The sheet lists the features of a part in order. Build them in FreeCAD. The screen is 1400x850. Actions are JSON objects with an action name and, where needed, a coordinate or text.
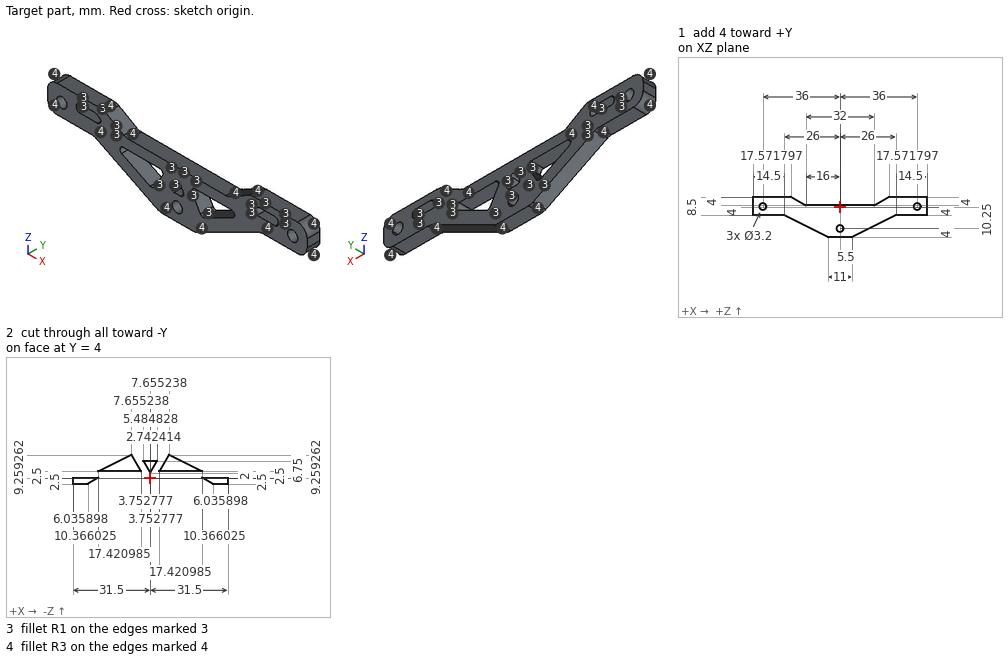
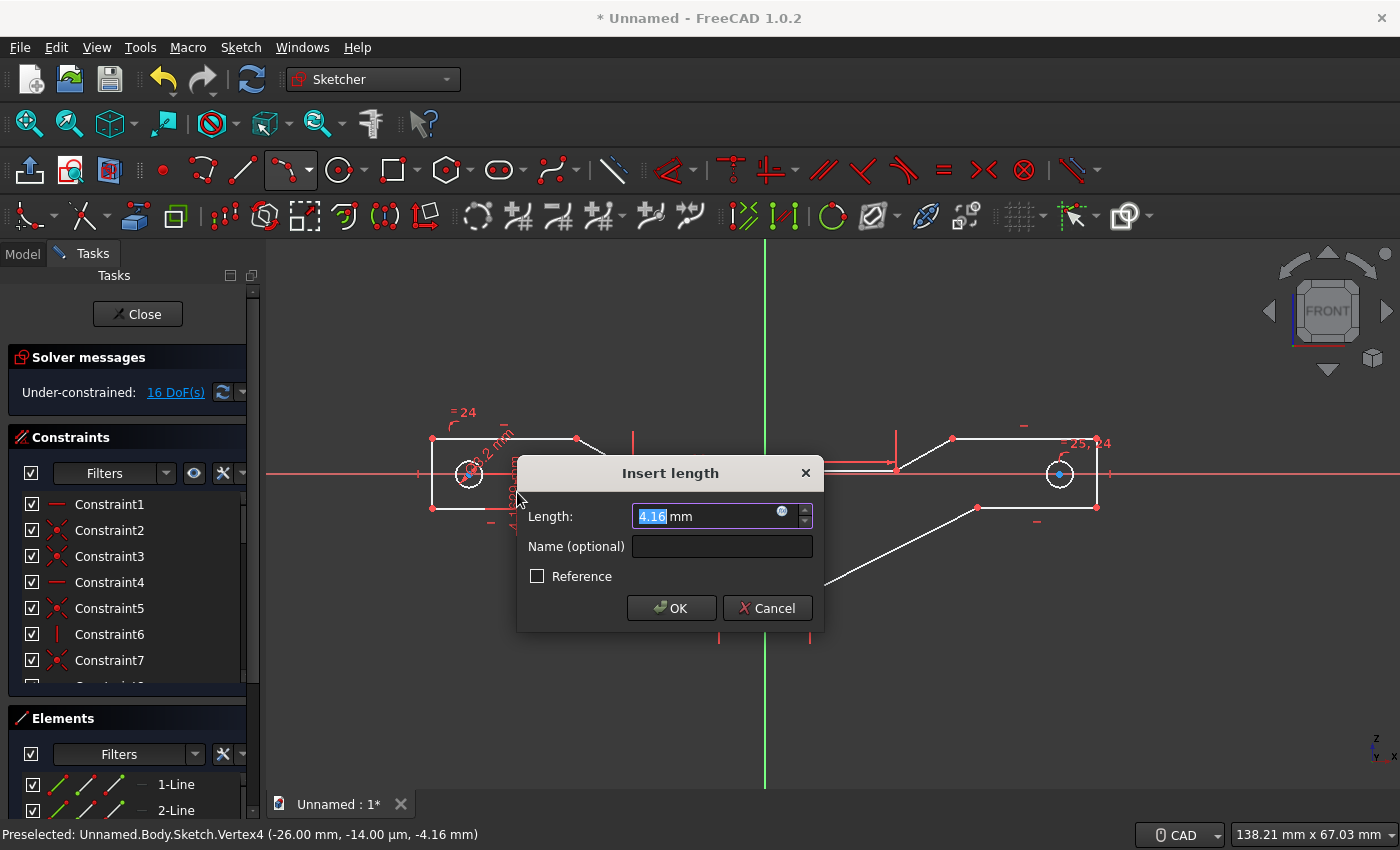
{"action": "type", "text": "4"}
{"action": "key", "text": "Return"}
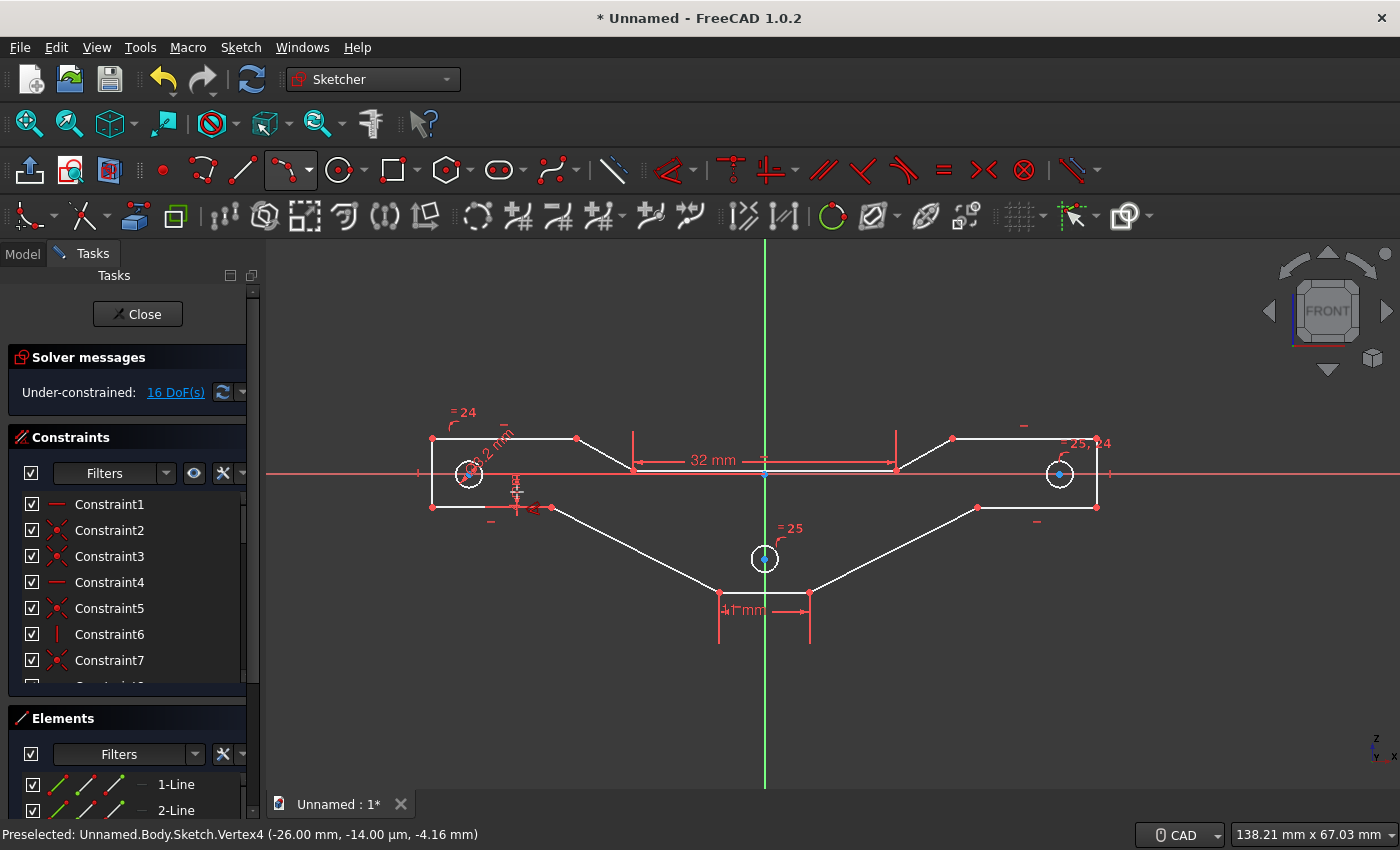
{"action": "left_click", "coordinate": [1097, 508]}
{"action": "left_click", "coordinate": [1131, 491]}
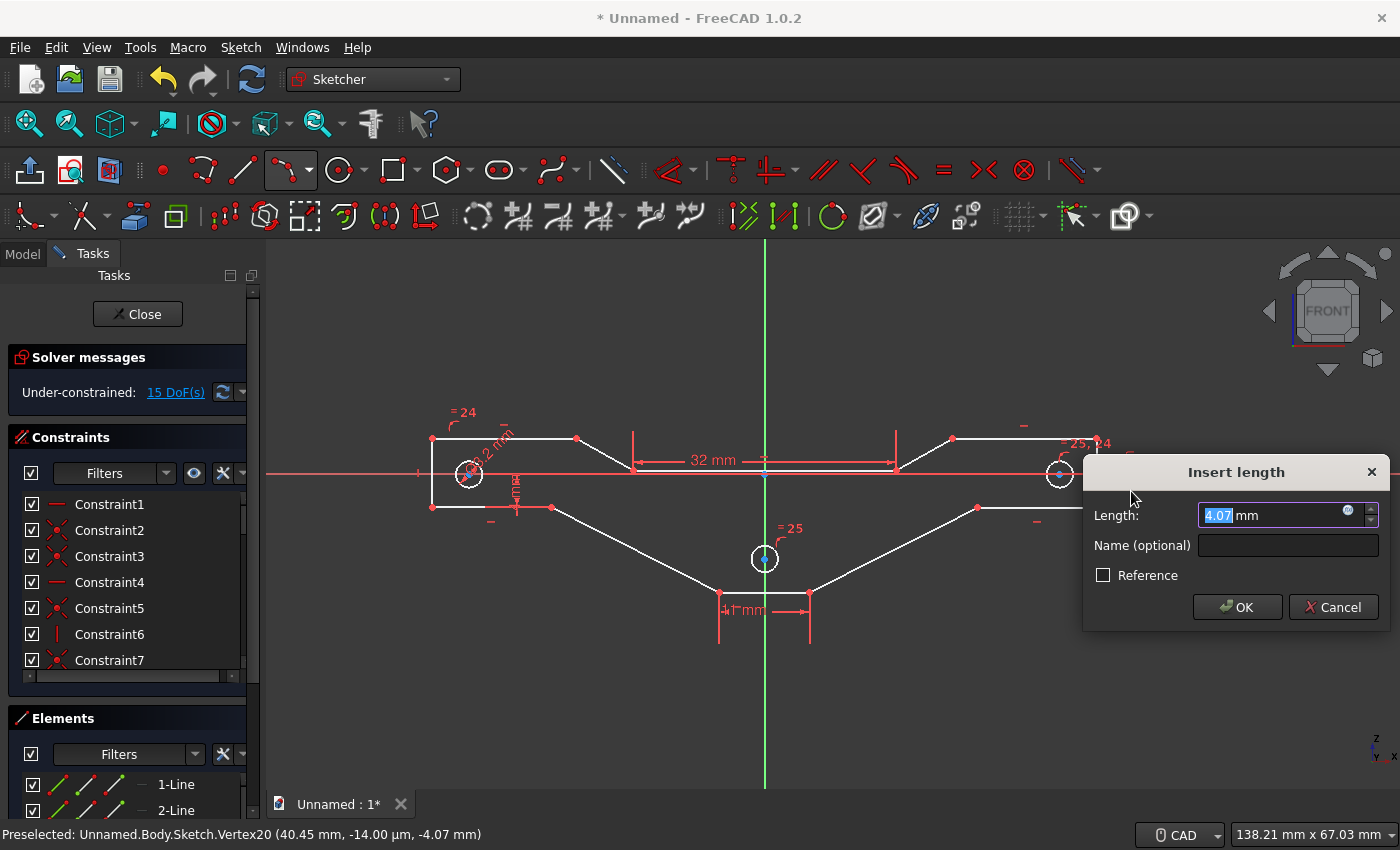
{"action": "type", "text": "4"}
{"action": "key", "text": "Return"}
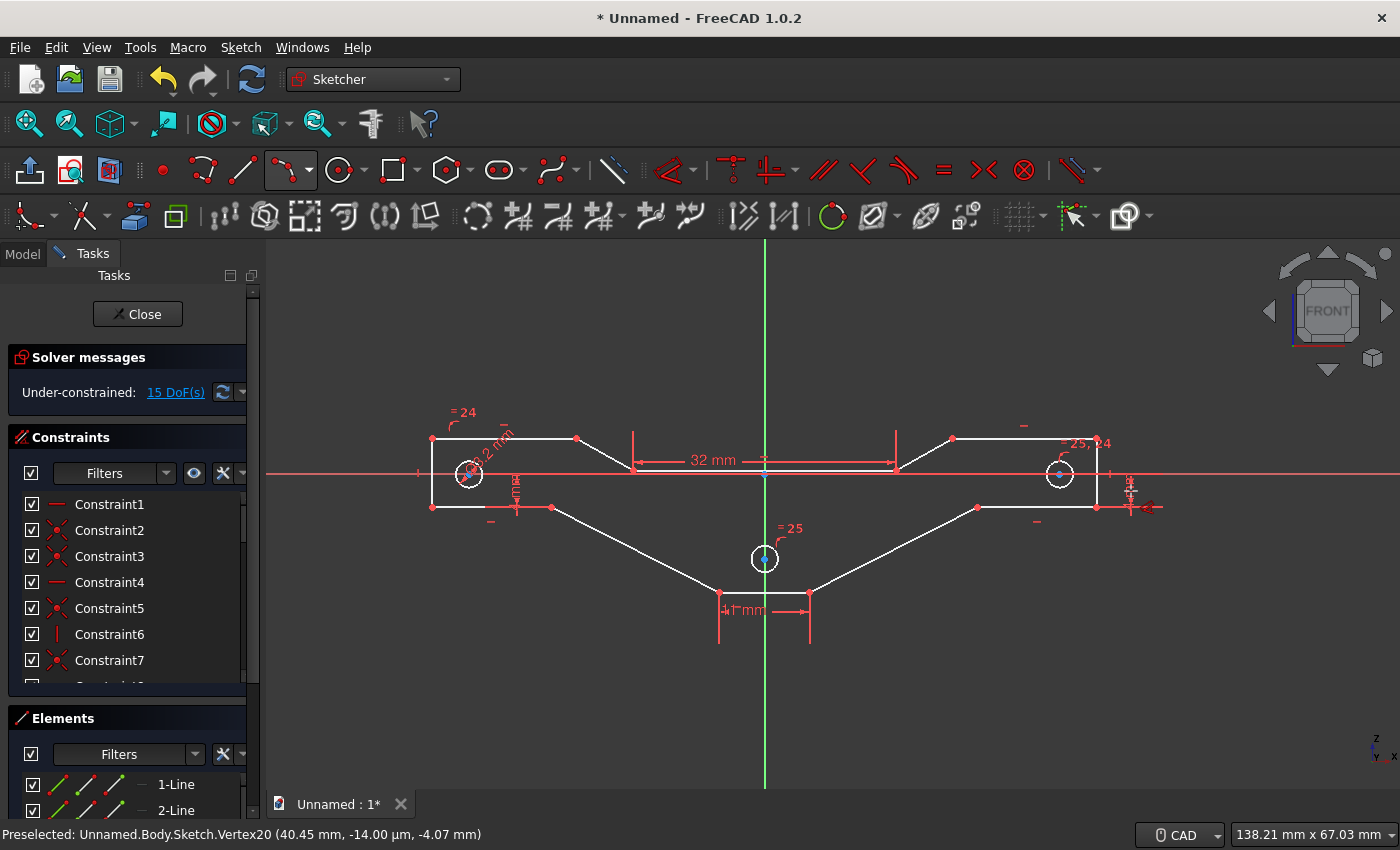
{"action": "left_click", "coordinate": [594, 448]}
{"action": "left_click", "coordinate": [787, 455]}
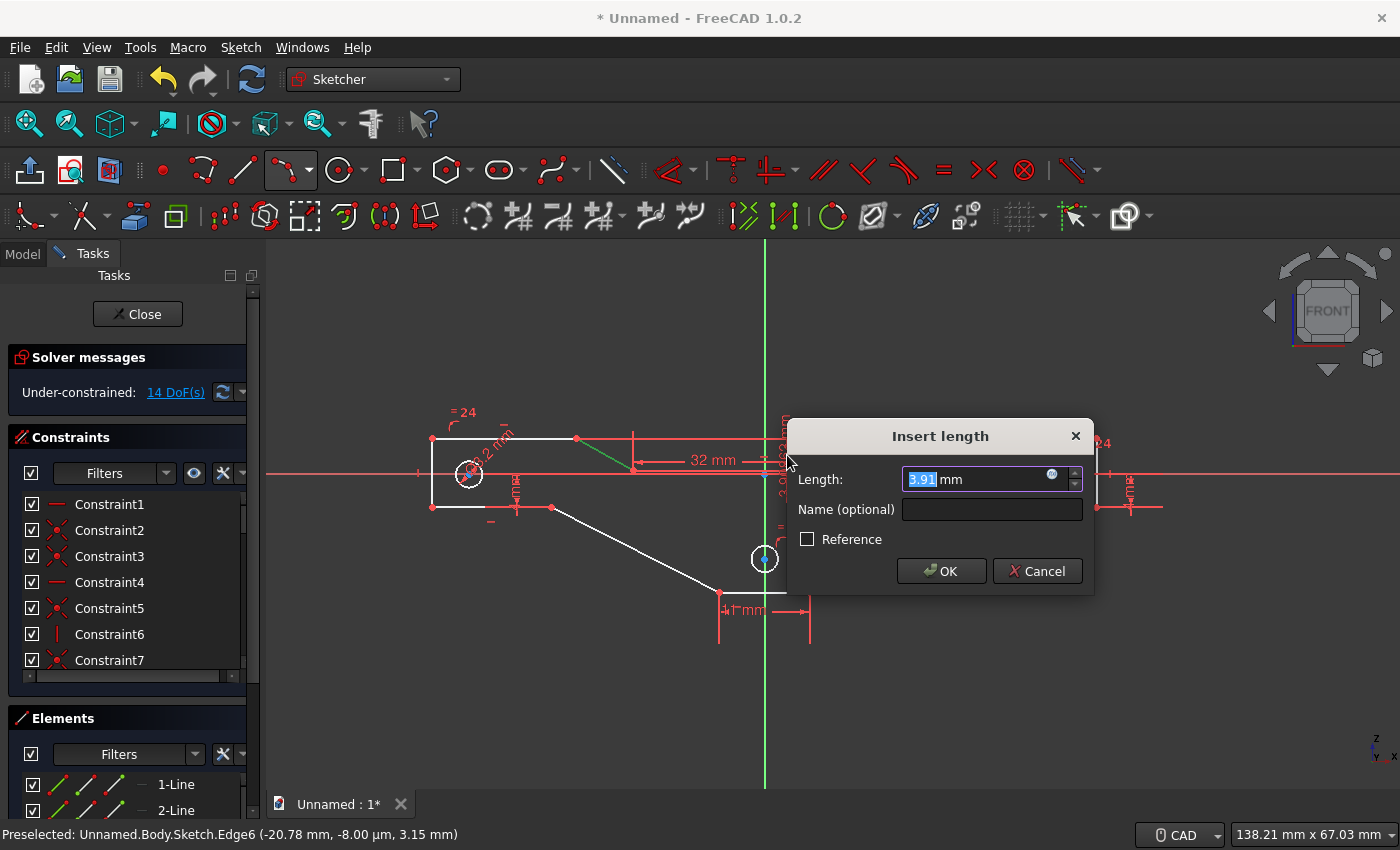
{"action": "type", "text": "4"}
{"action": "key", "text": "Return"}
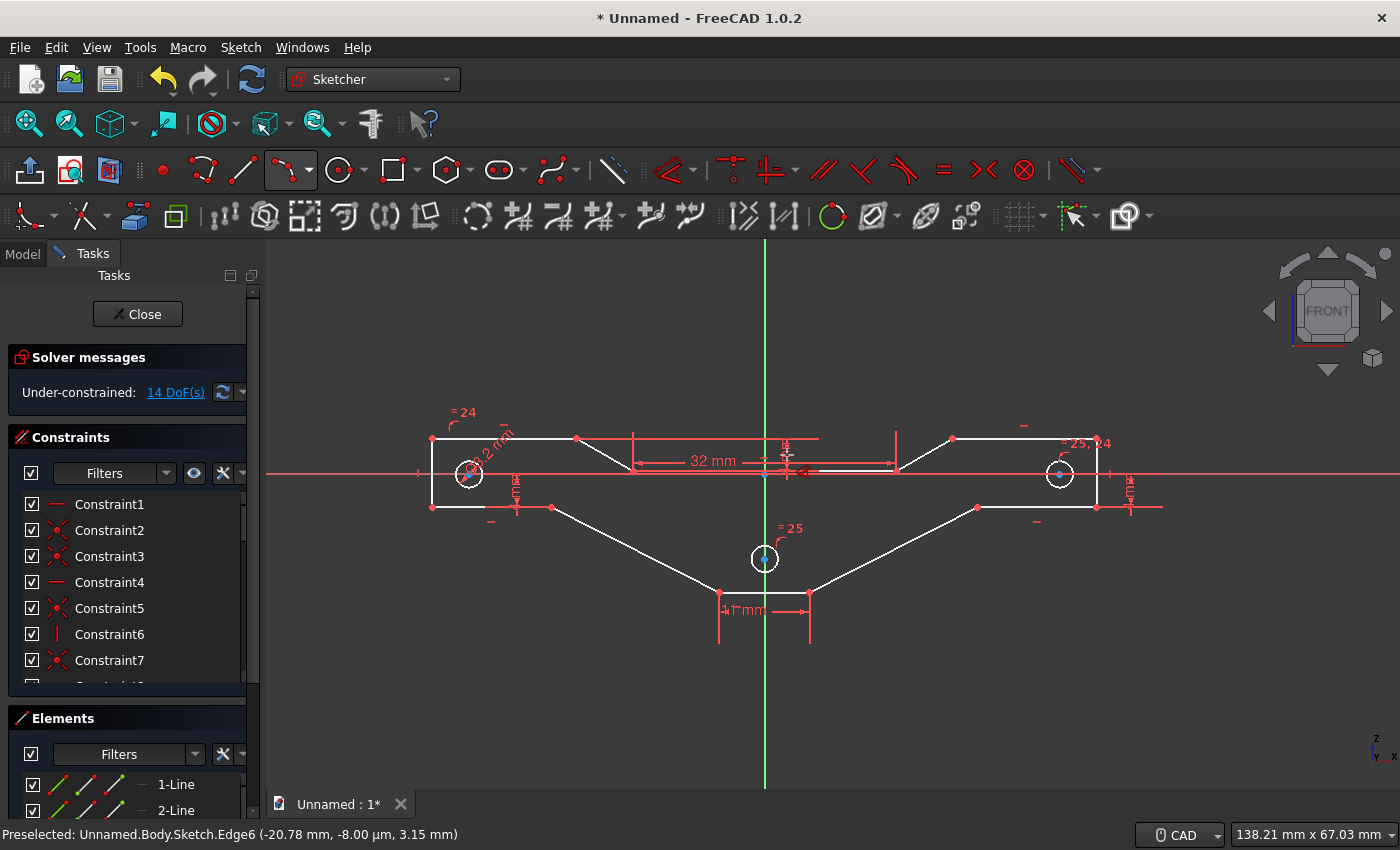
{"action": "left_click", "coordinate": [913, 462]}
{"action": "left_click", "coordinate": [987, 455]}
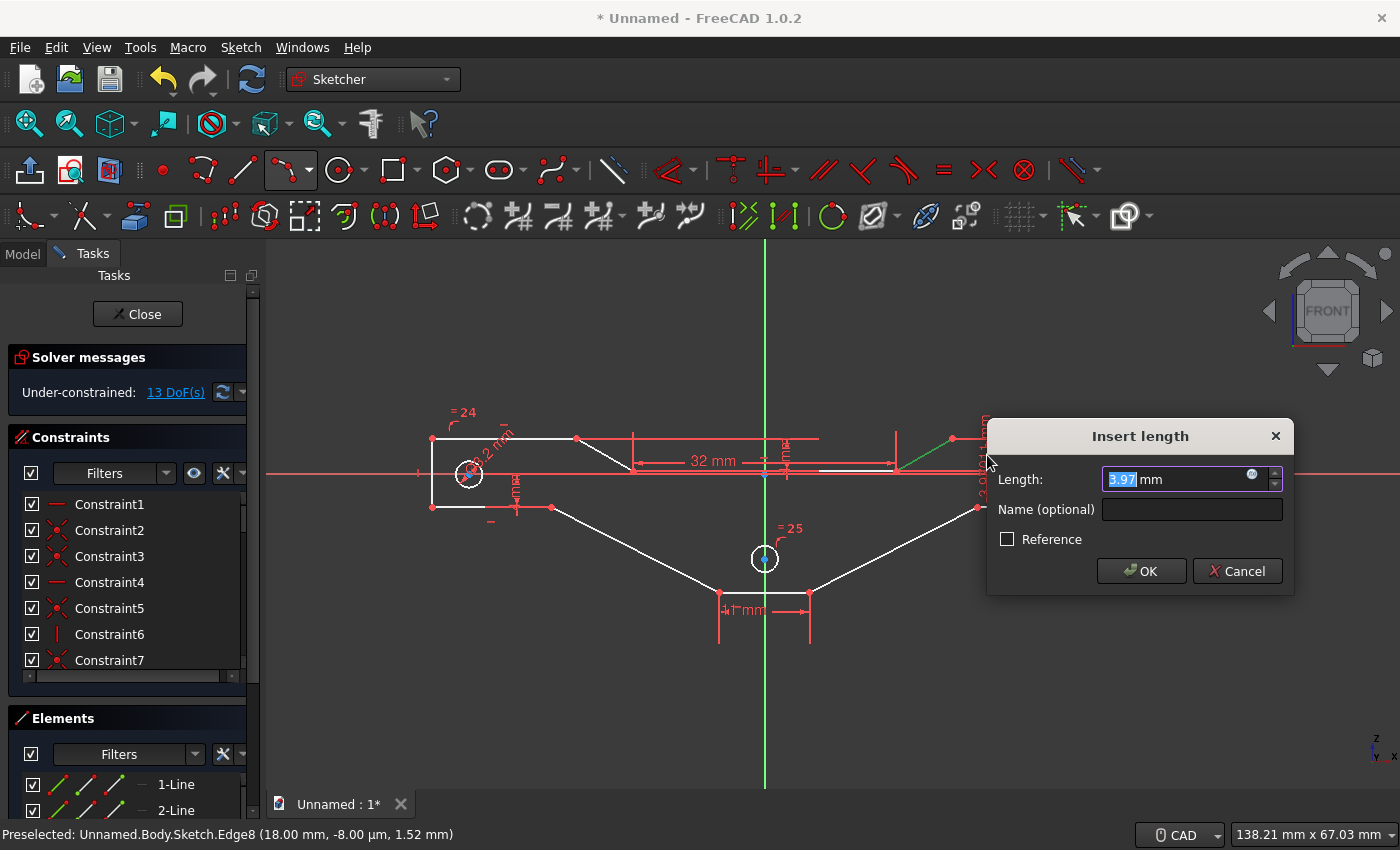
{"action": "type", "text": "4"}
{"action": "key", "text": "Return"}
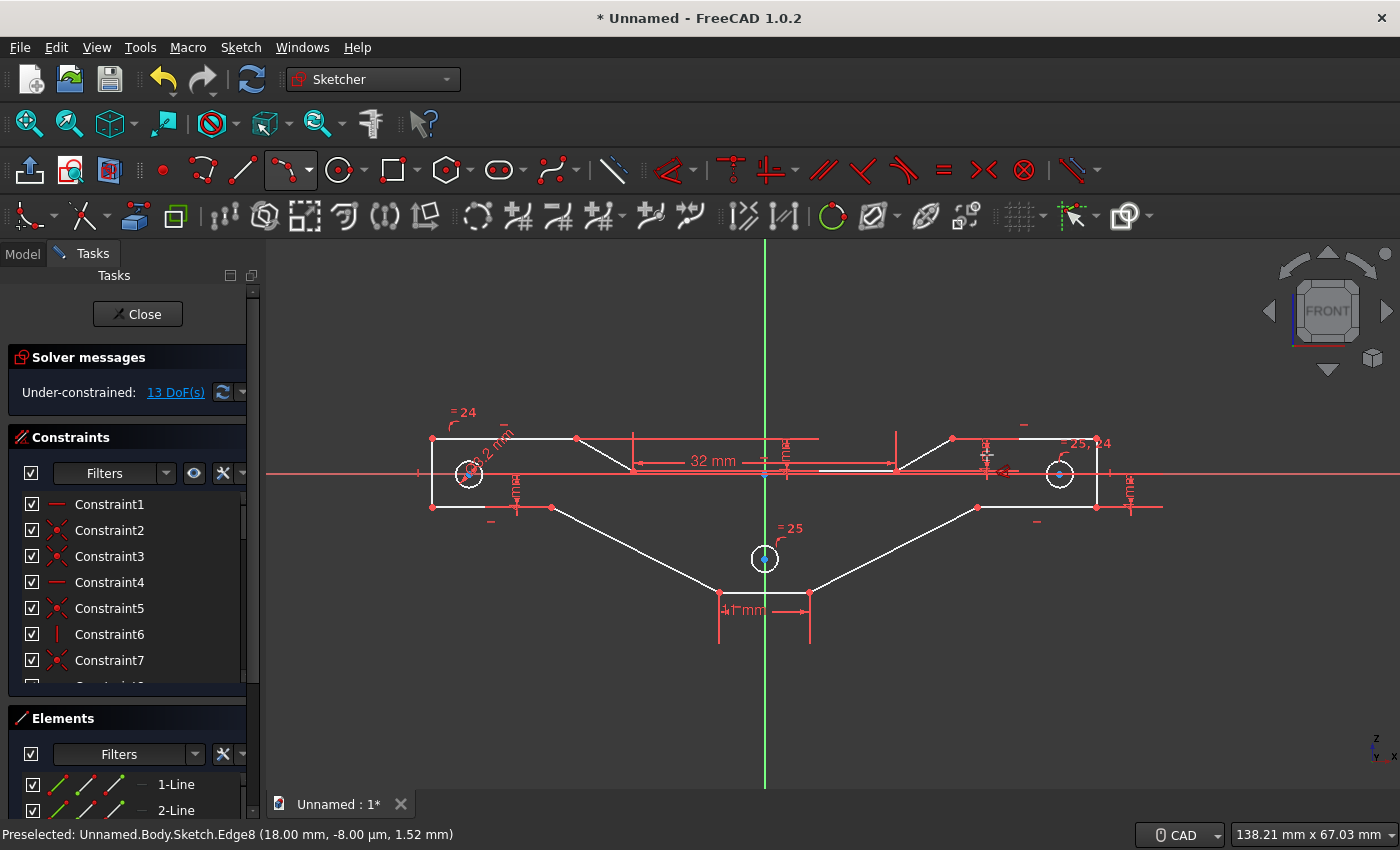
{"action": "left_click", "coordinate": [469, 474]}
{"action": "left_click", "coordinate": [617, 440]}